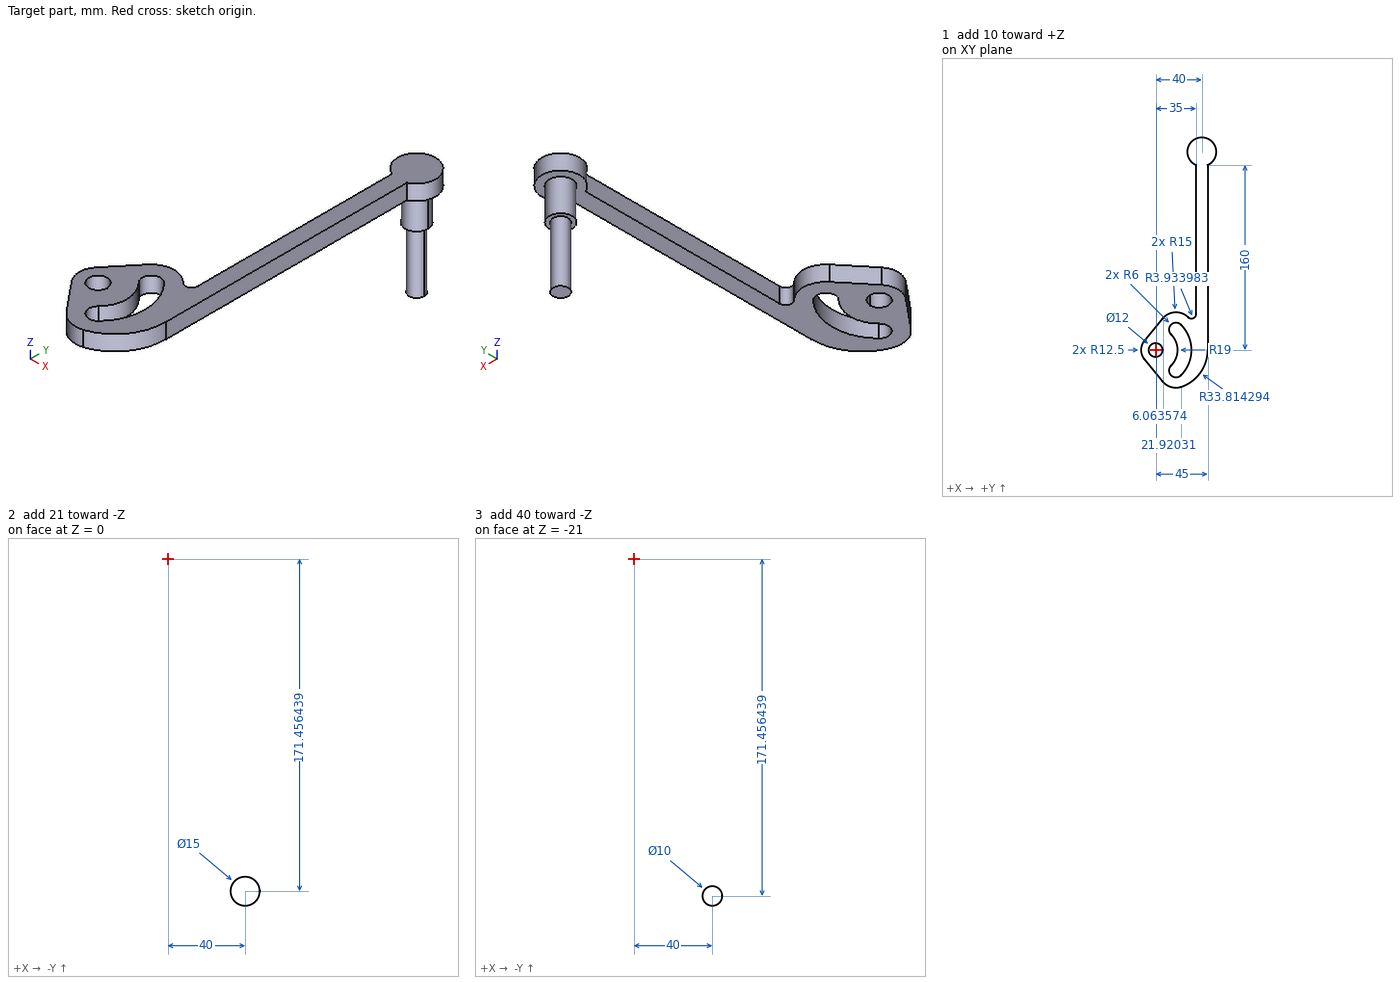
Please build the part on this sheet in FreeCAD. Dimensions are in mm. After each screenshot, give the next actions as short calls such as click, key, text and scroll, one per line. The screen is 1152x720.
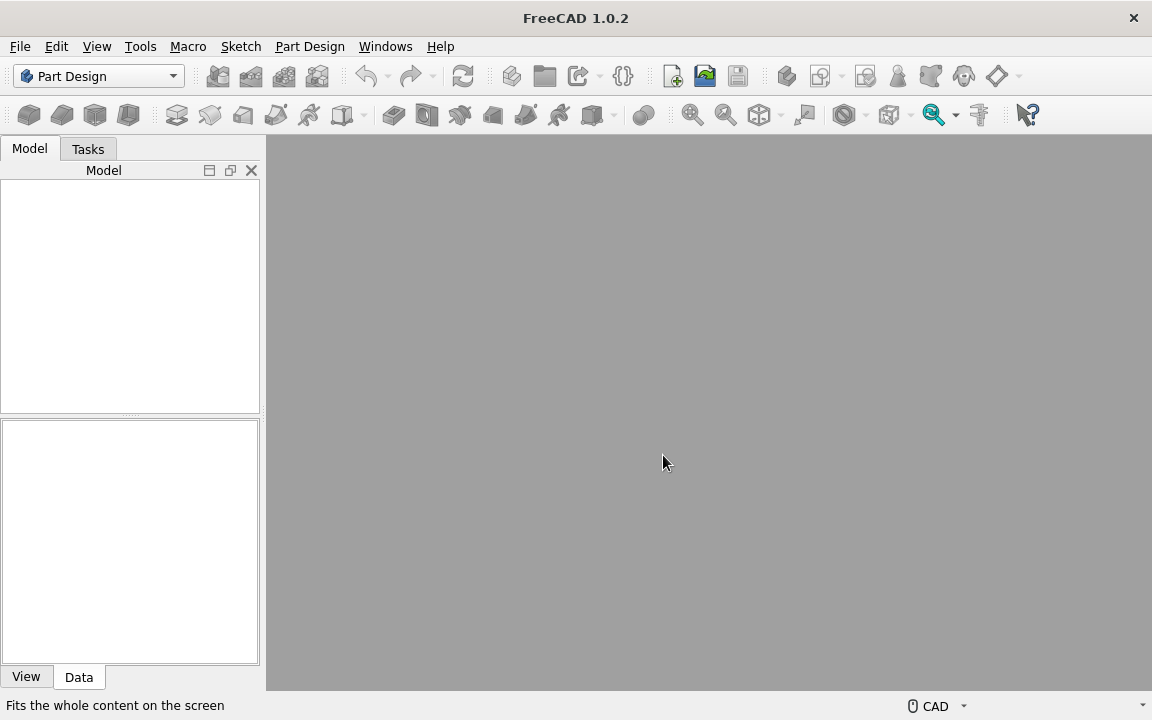
key(ctrl+n)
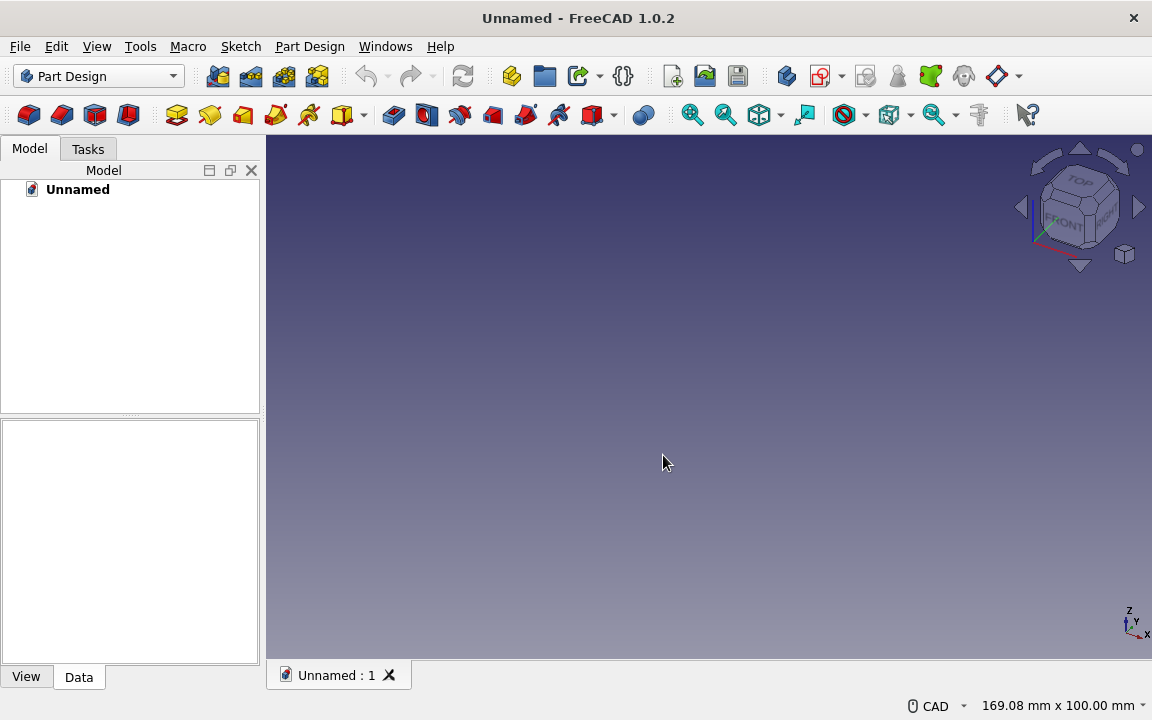
click(820, 76)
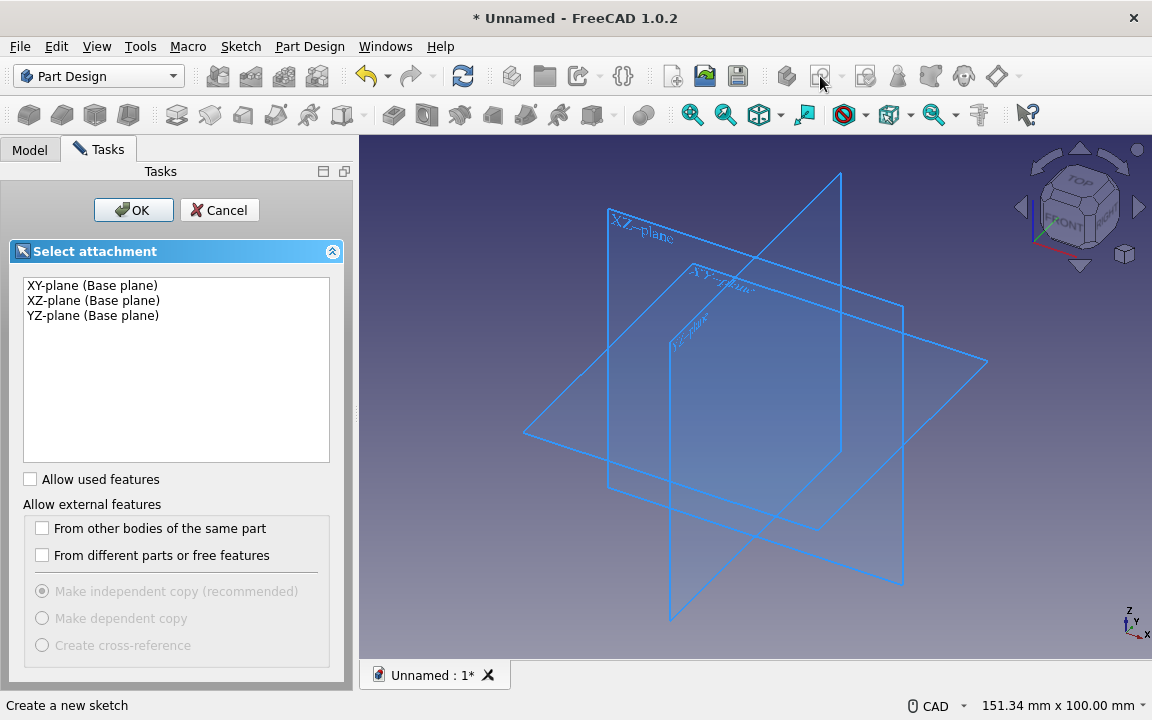
click(84, 286)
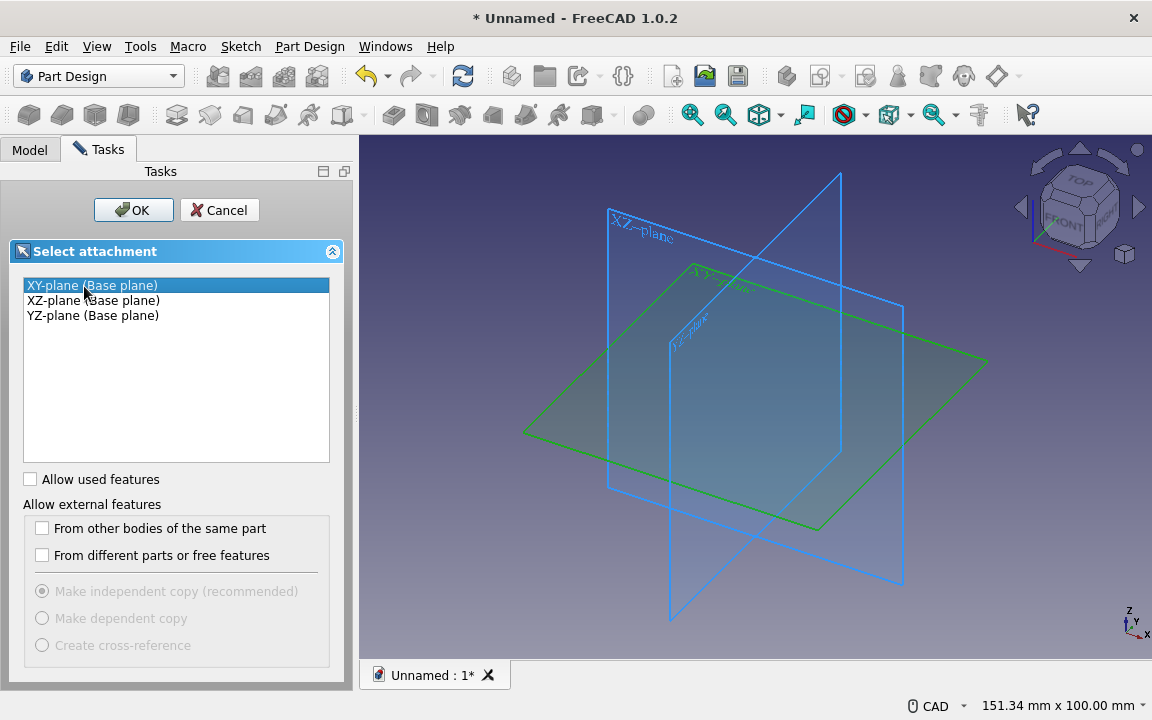
click(134, 210)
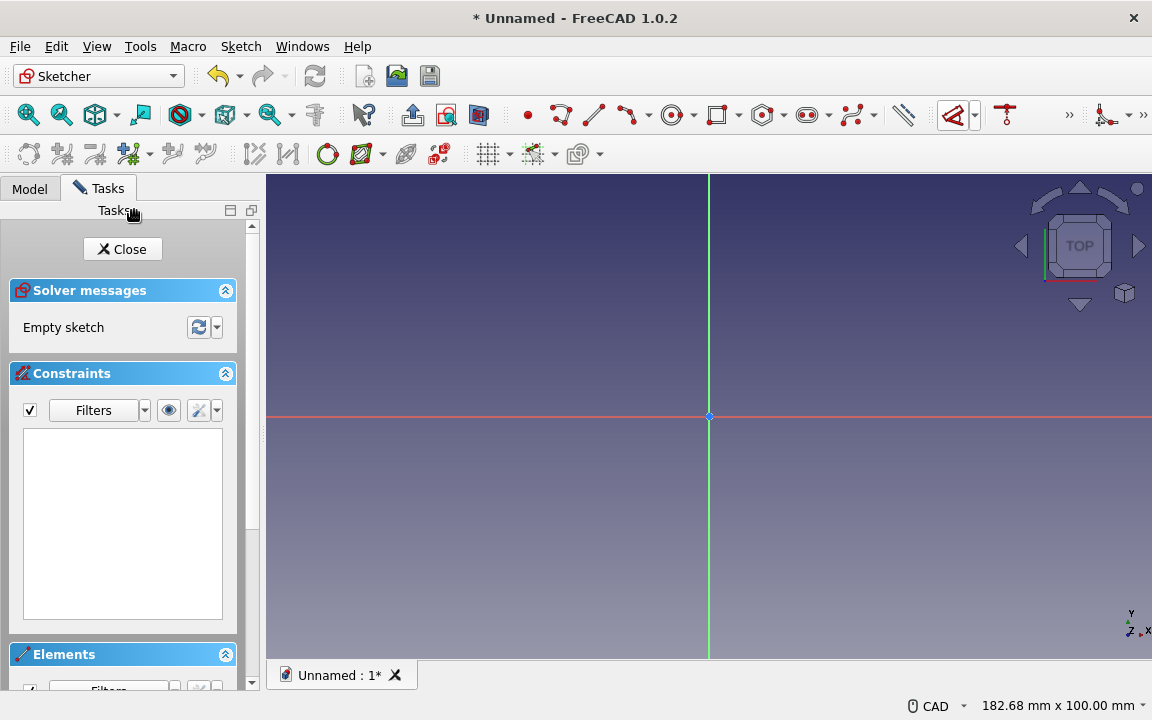
scroll(577, 575, down, 6)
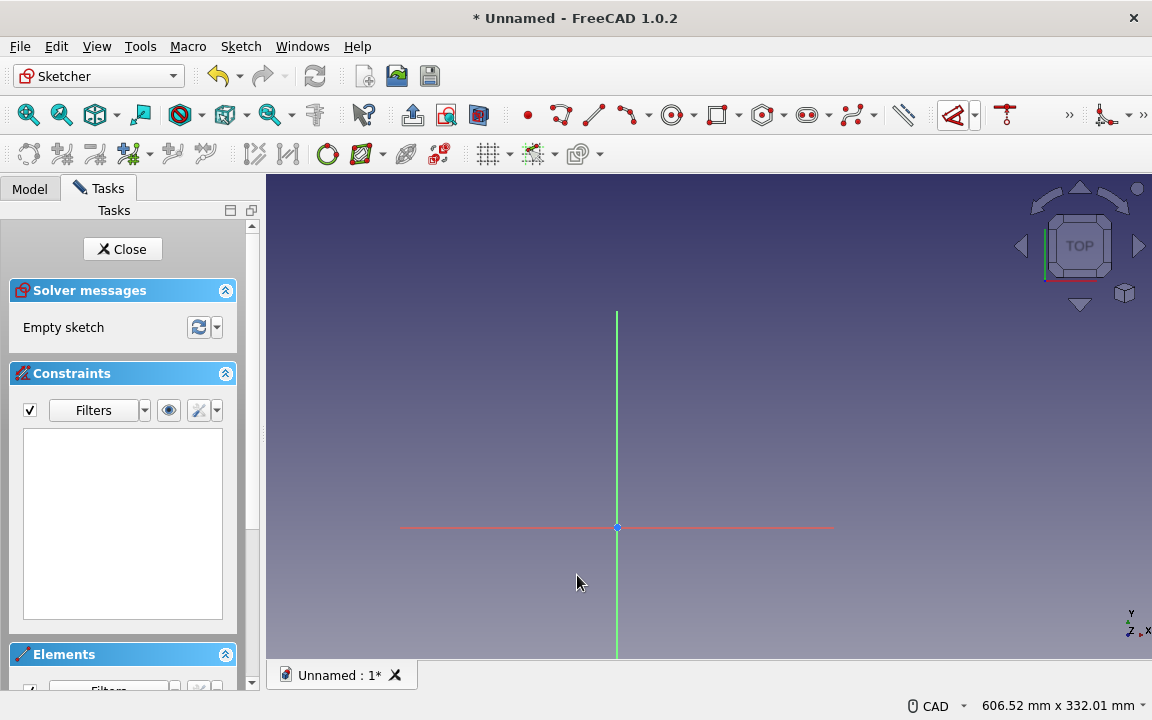
key(g)
key(l)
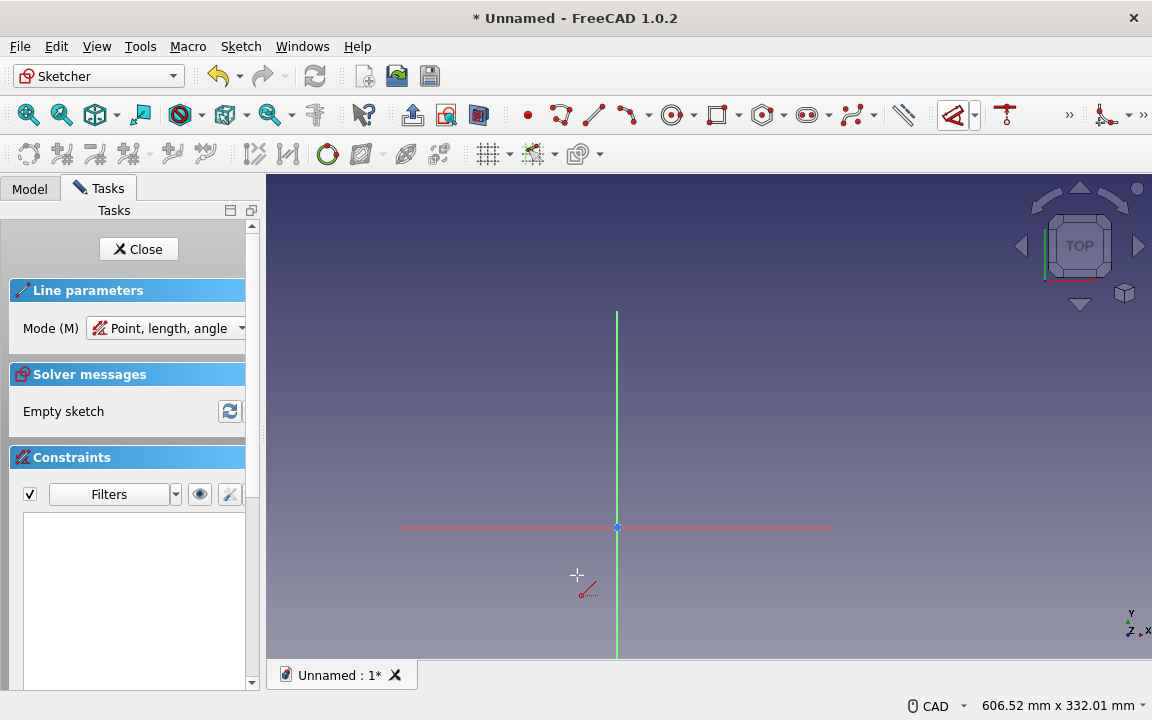
scroll(626, 488, up, 3)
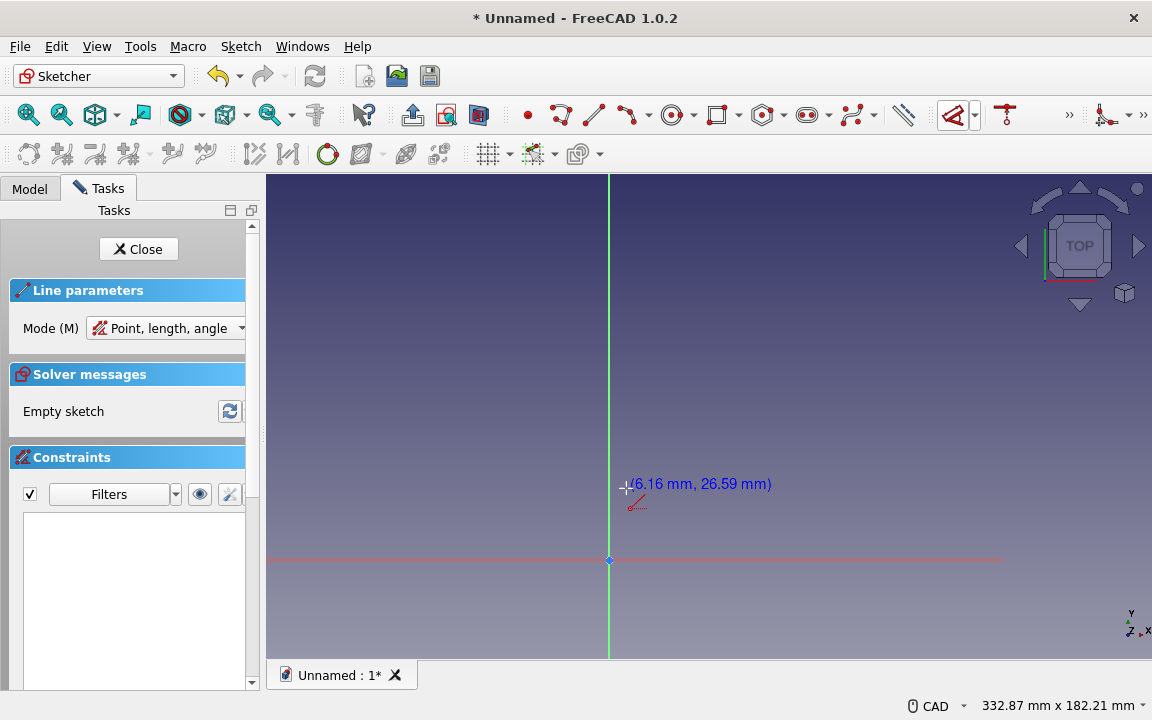
click(625, 488)
click(584, 539)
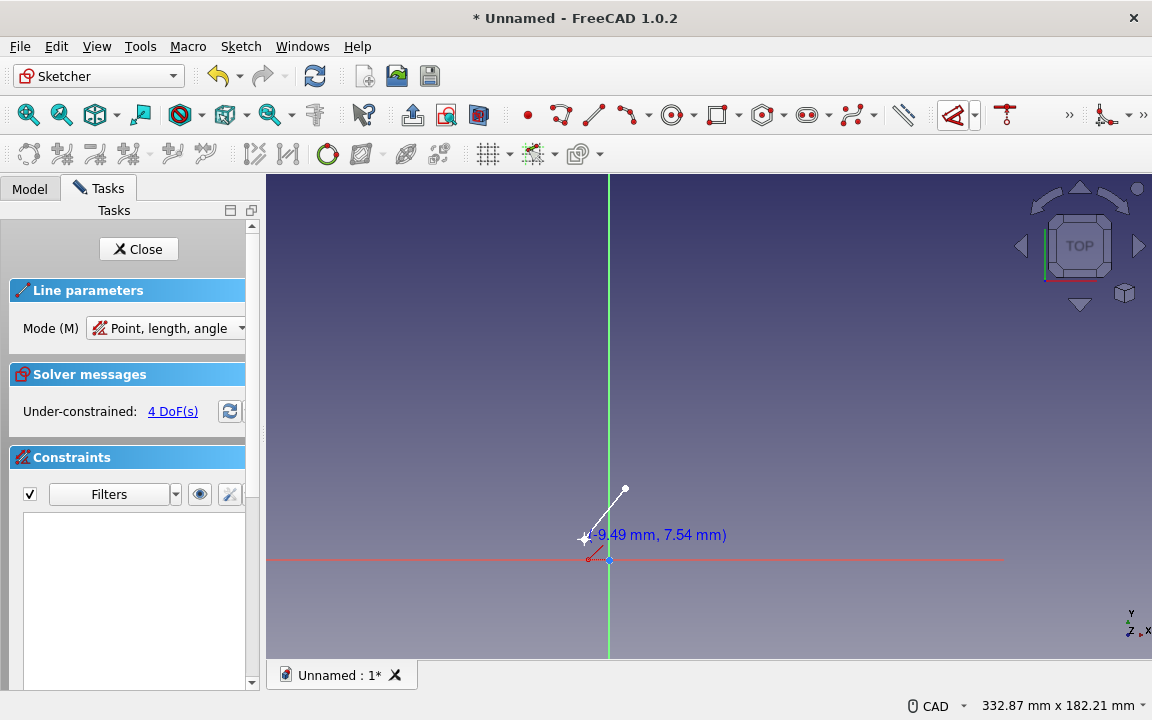
click(584, 581)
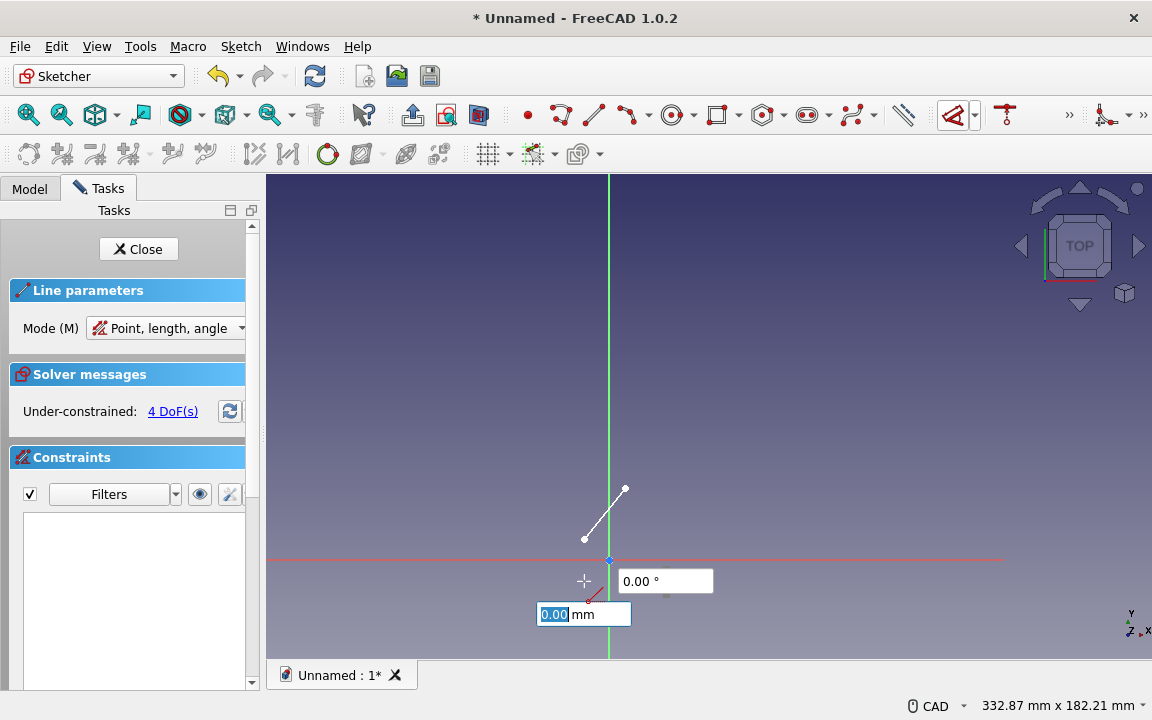
scroll(626, 488, down, 3)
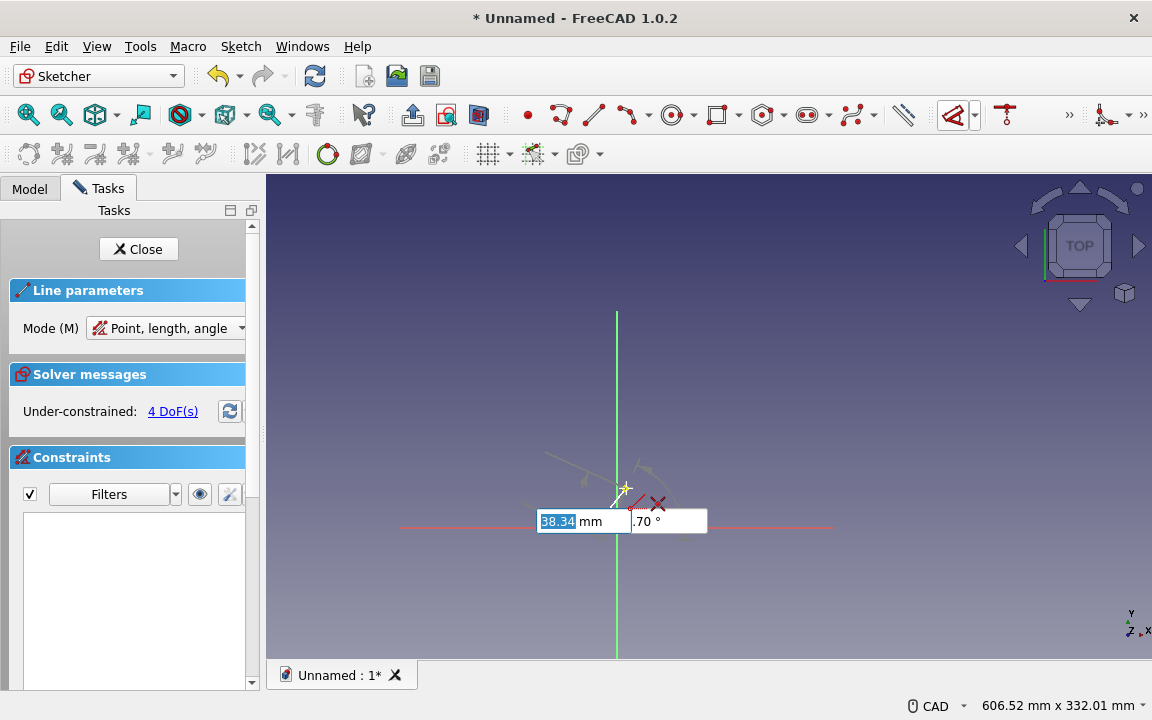
scroll(626, 568, up, 3)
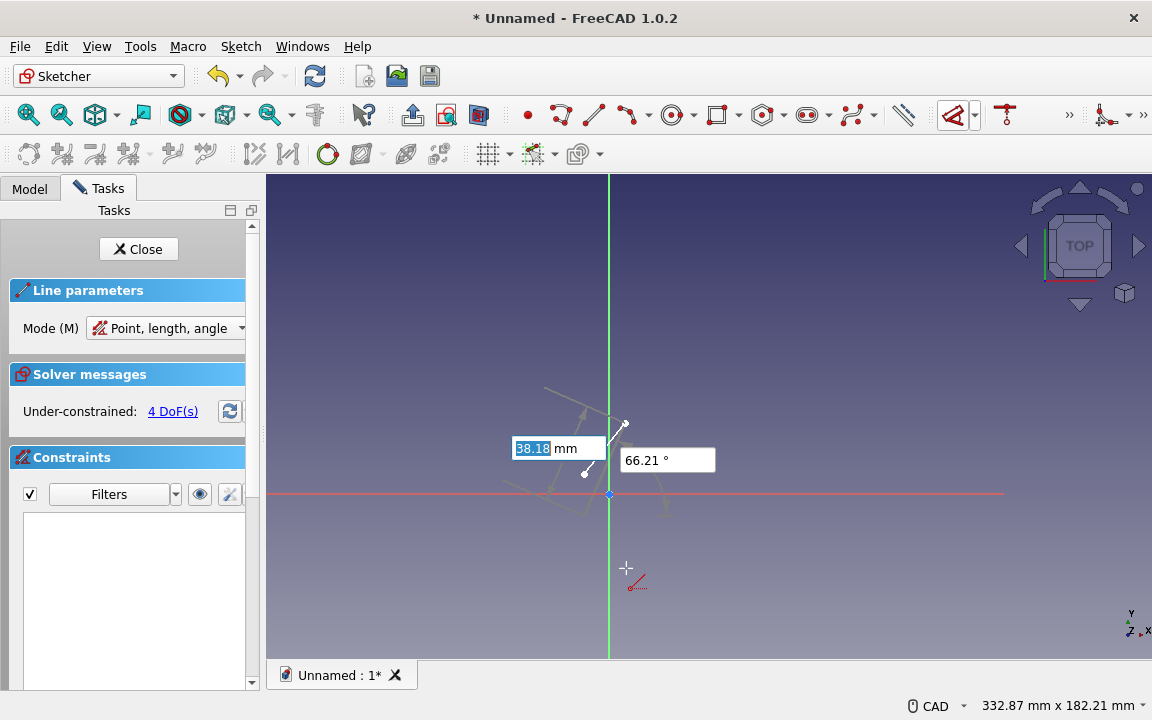
click(625, 566)